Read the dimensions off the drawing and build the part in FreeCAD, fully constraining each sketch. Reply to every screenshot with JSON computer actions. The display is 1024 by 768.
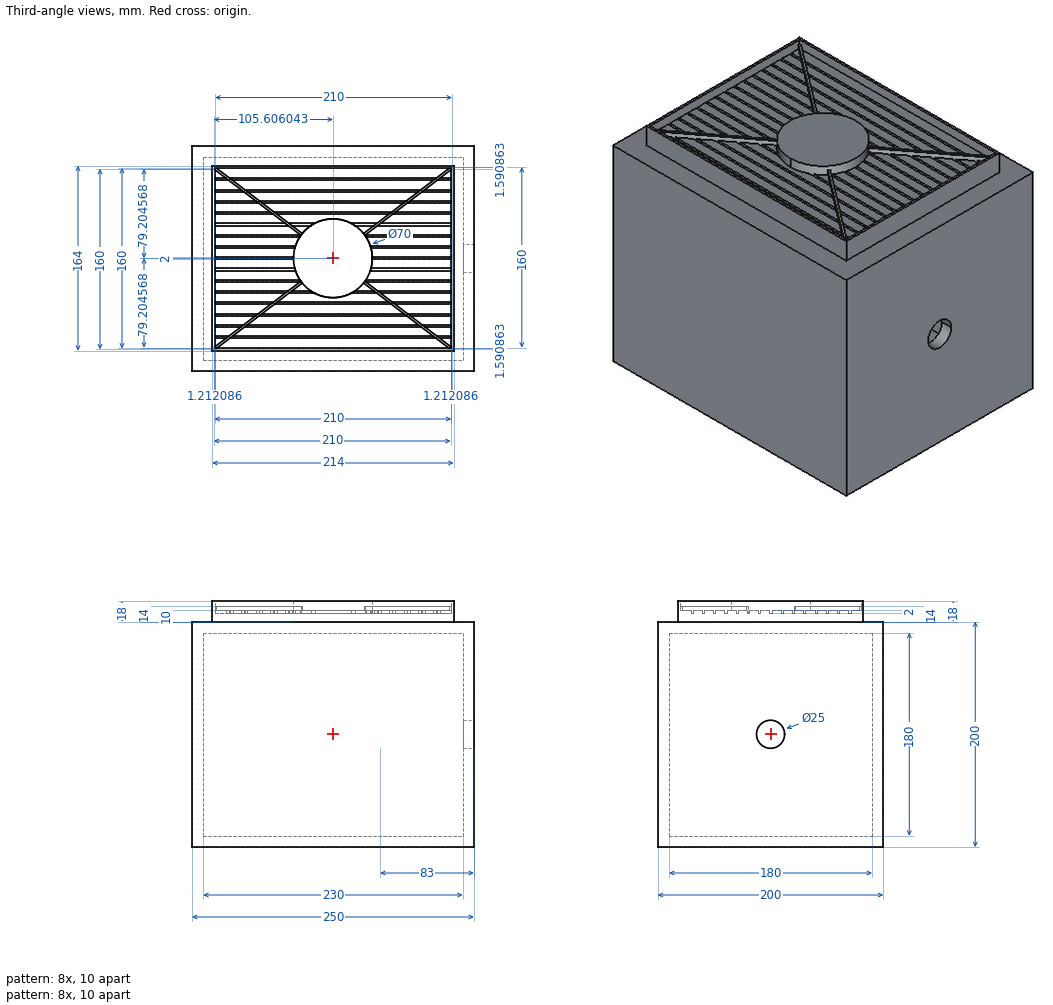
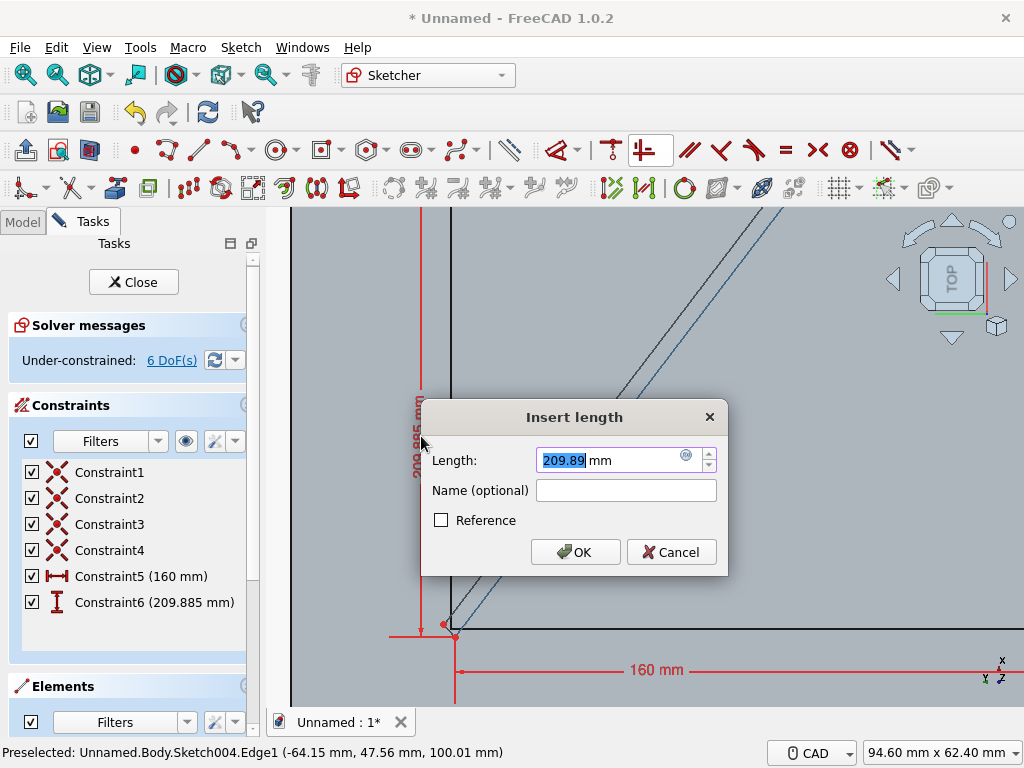
{"action": "type", "text": "210"}
{"action": "key", "text": "Return"}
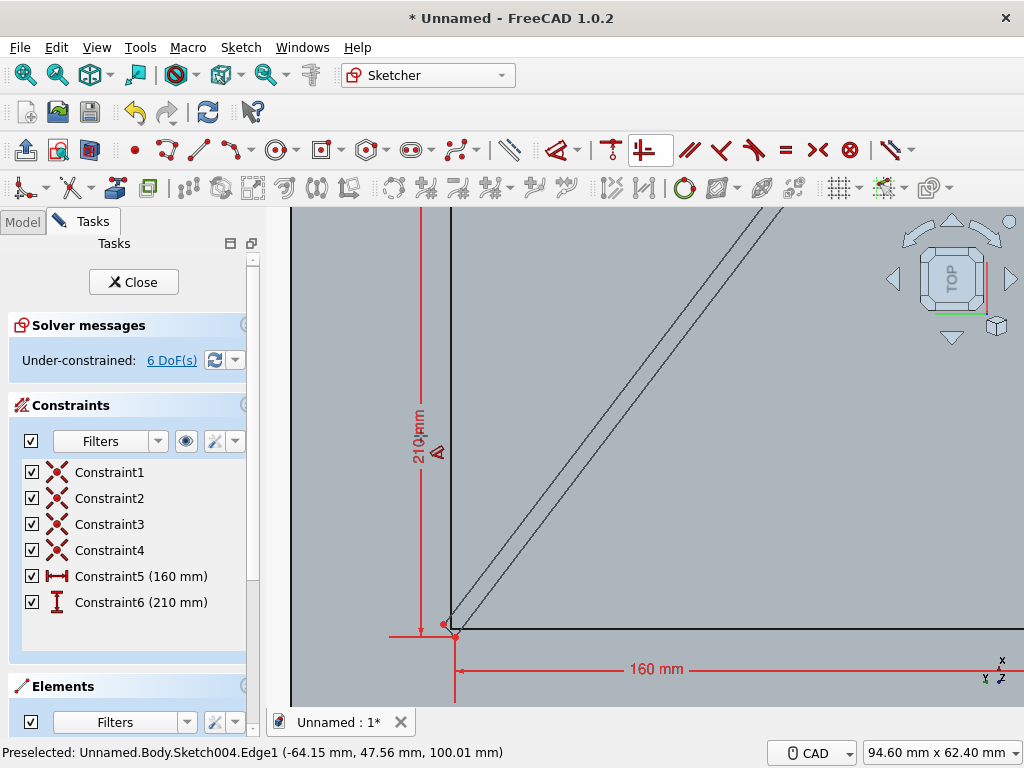
{"action": "left_click", "coordinate": [701, 289]}
{"action": "left_click", "coordinate": [556, 659]}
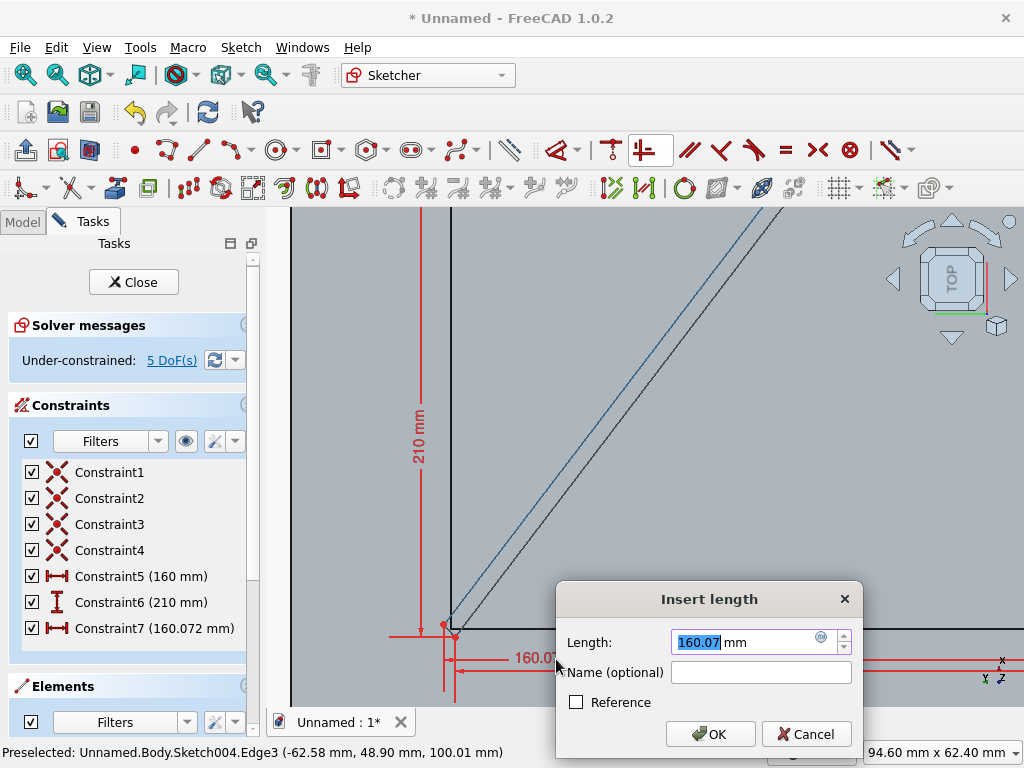
{"action": "type", "text": "160"}
{"action": "key", "text": "Return"}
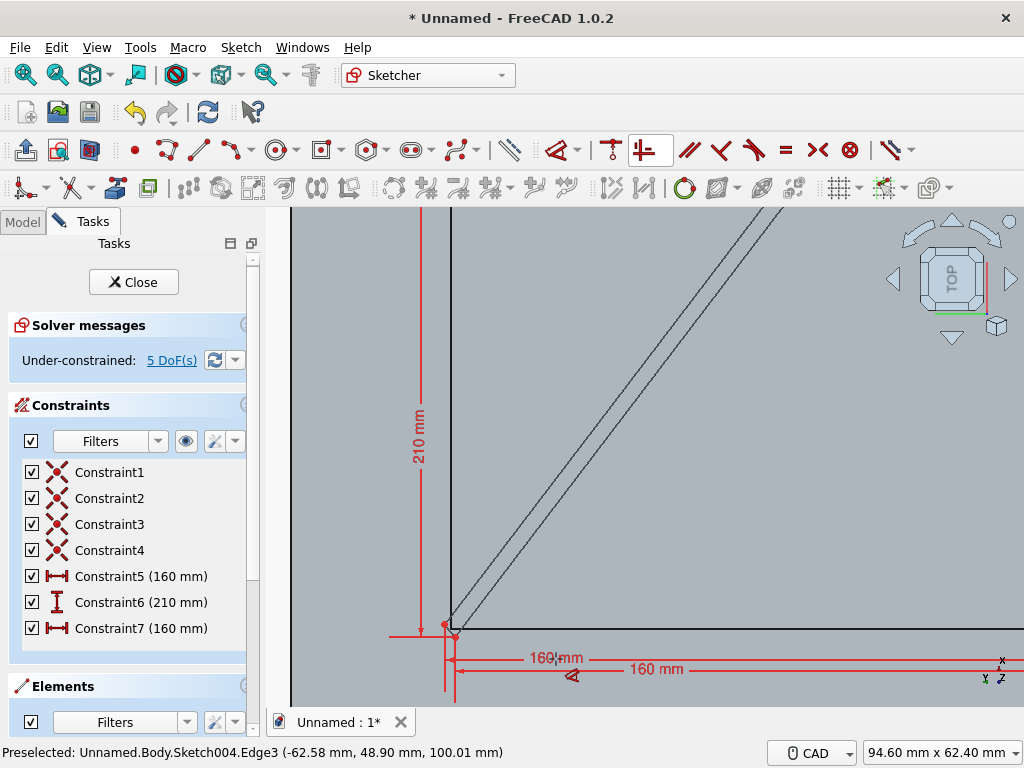
{"action": "left_click", "coordinate": [701, 289]}
{"action": "left_click", "coordinate": [411, 340]}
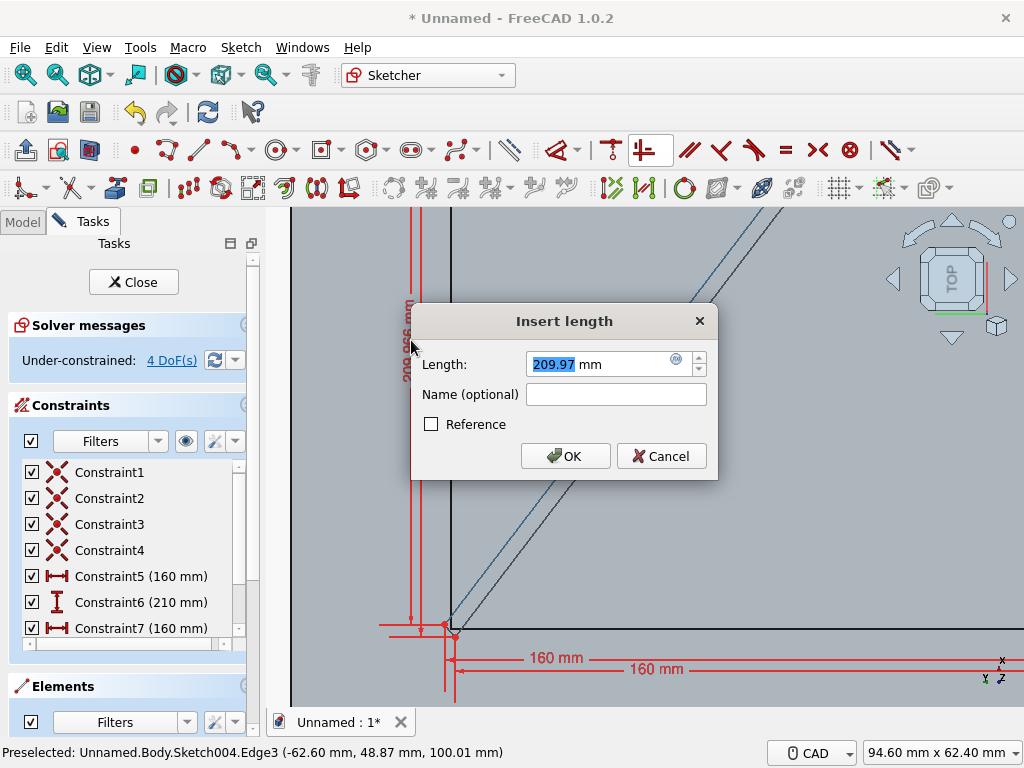
{"action": "type", "text": "210"}
{"action": "key", "text": "Return"}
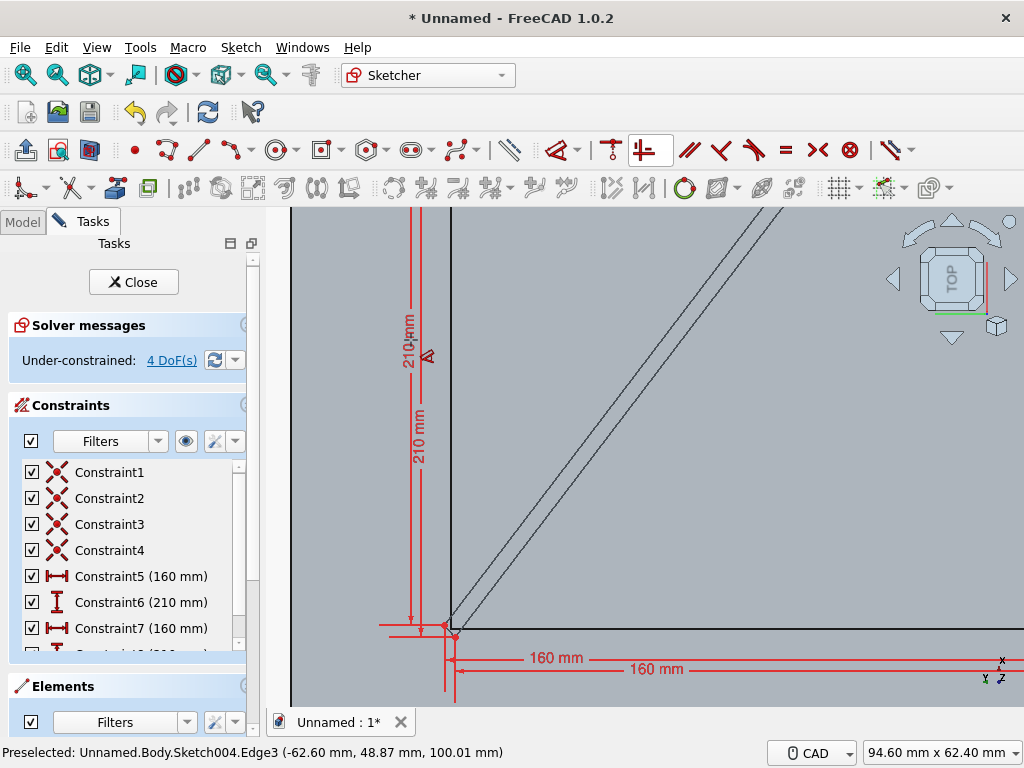
{"action": "scroll", "coordinate": [446, 626], "scroll_direction": "down", "scroll_amount": 8}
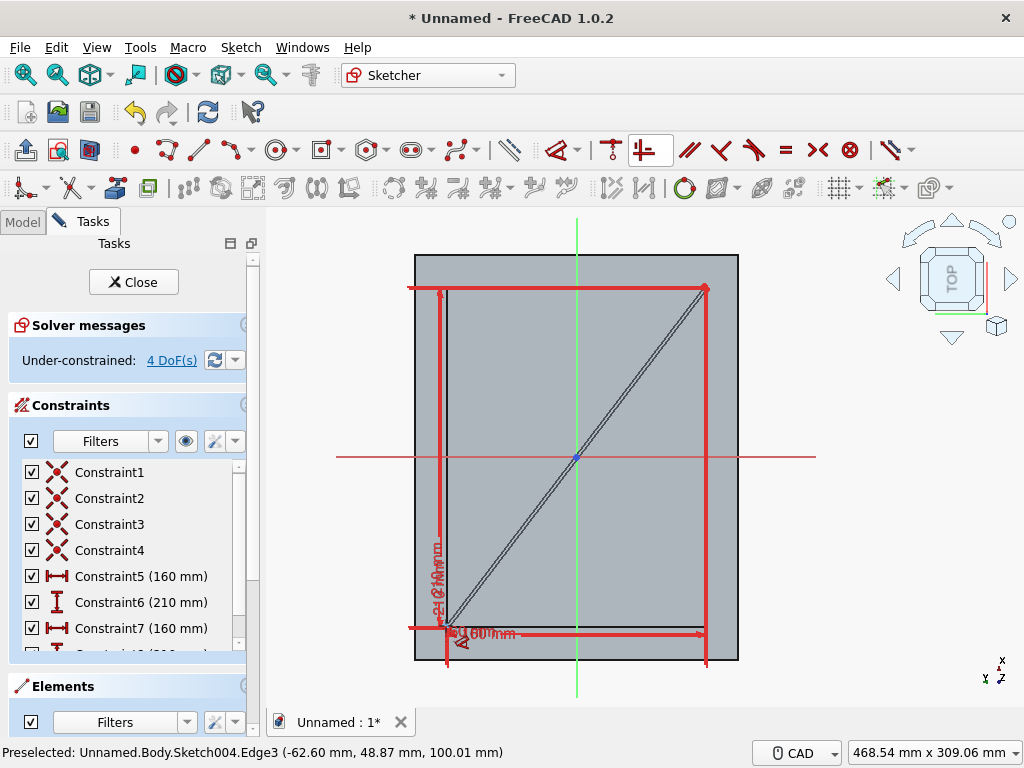
{"action": "scroll", "coordinate": [706, 288], "scroll_direction": "up", "scroll_amount": 14}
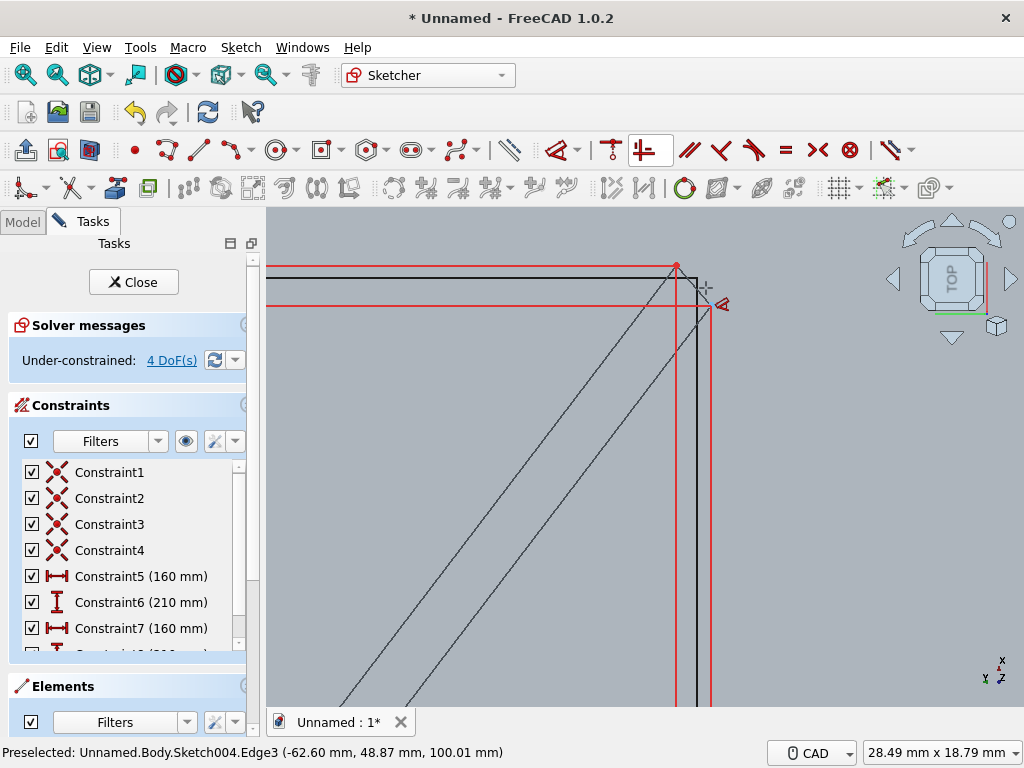
{"action": "left_click", "coordinate": [694, 286]}
{"action": "left_click", "coordinate": [702, 340]}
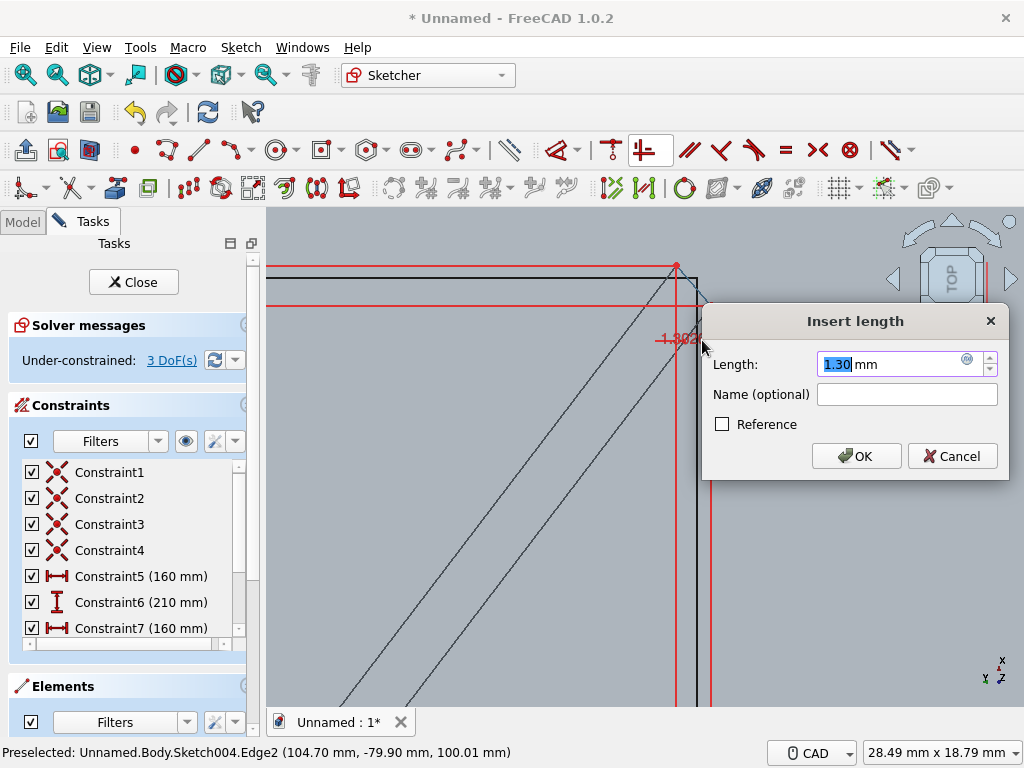
{"action": "type", "text": "1.590863"}
{"action": "key", "text": "Return"}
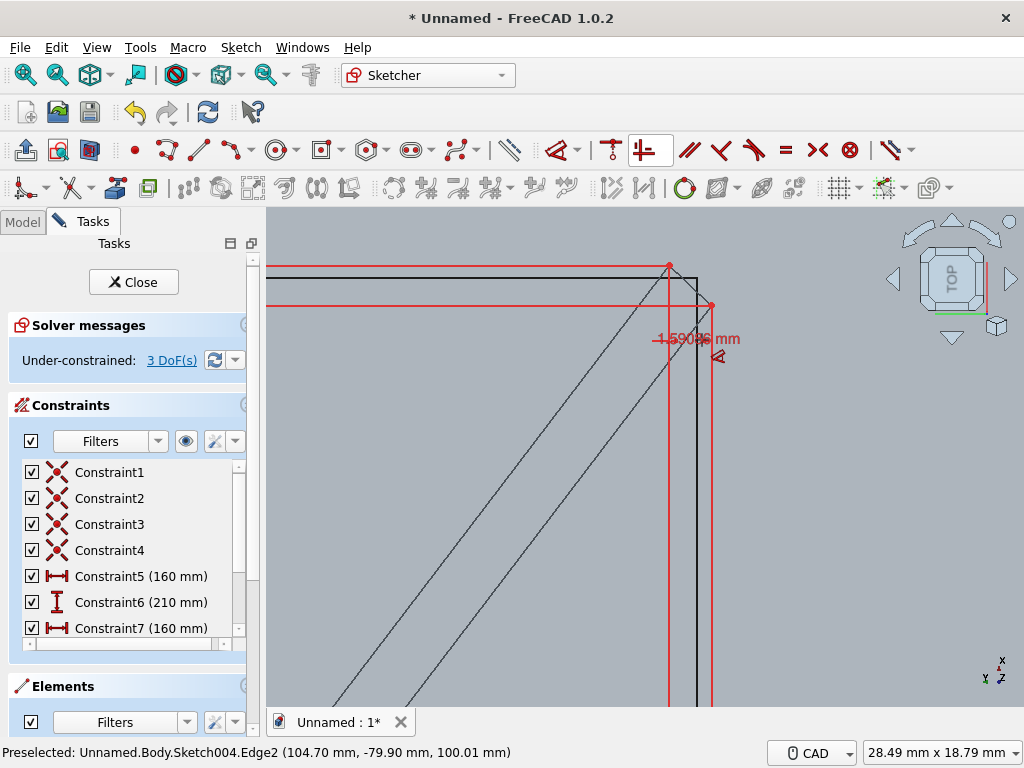
{"action": "scroll", "coordinate": [699, 294], "scroll_direction": "up", "scroll_amount": 2}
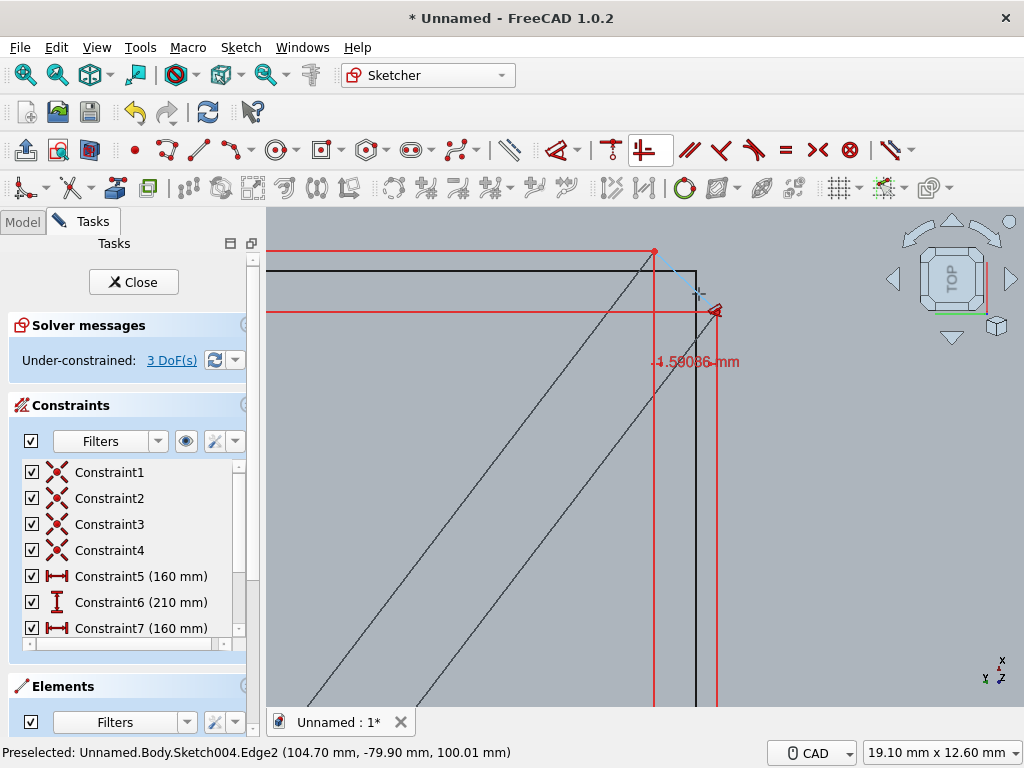
{"action": "left_click", "coordinate": [698, 294]}
{"action": "left_click", "coordinate": [751, 282]}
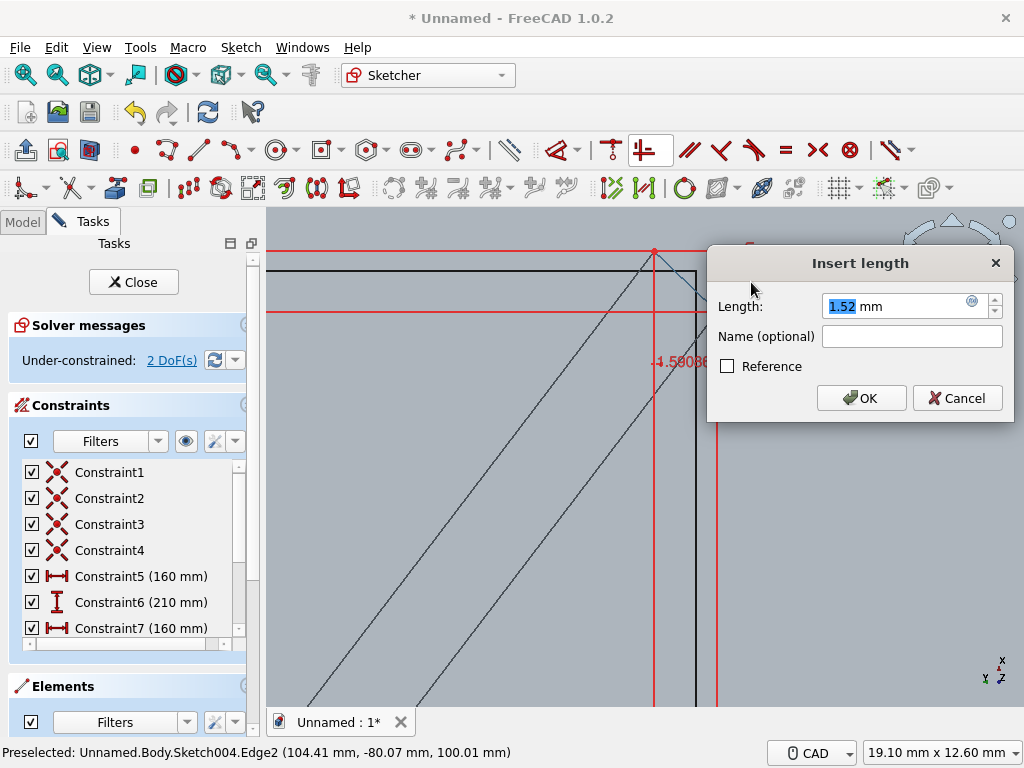
{"action": "type", "text": "1.212086"}
{"action": "key", "text": "Return"}